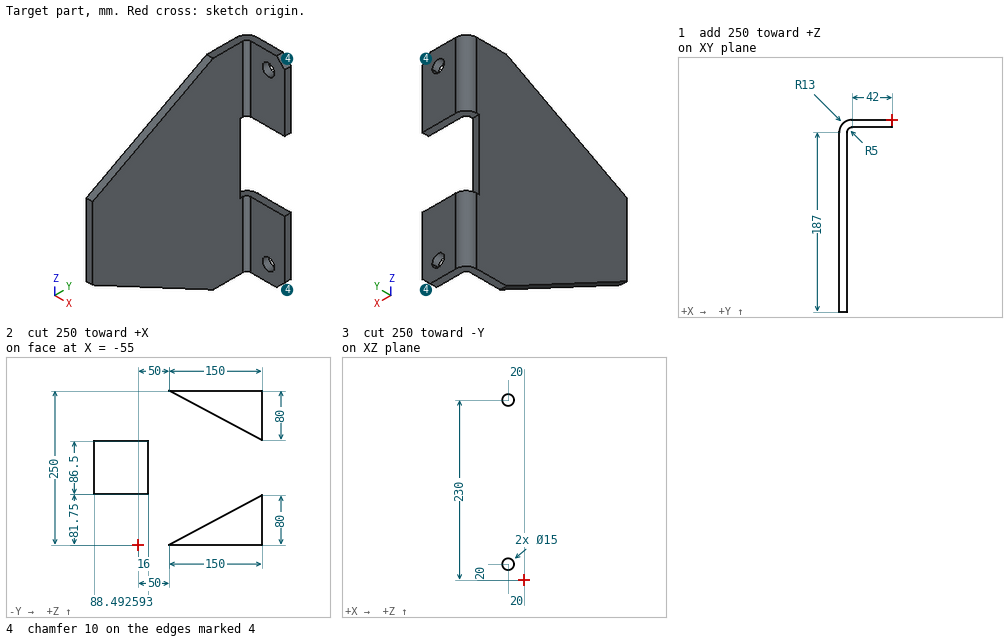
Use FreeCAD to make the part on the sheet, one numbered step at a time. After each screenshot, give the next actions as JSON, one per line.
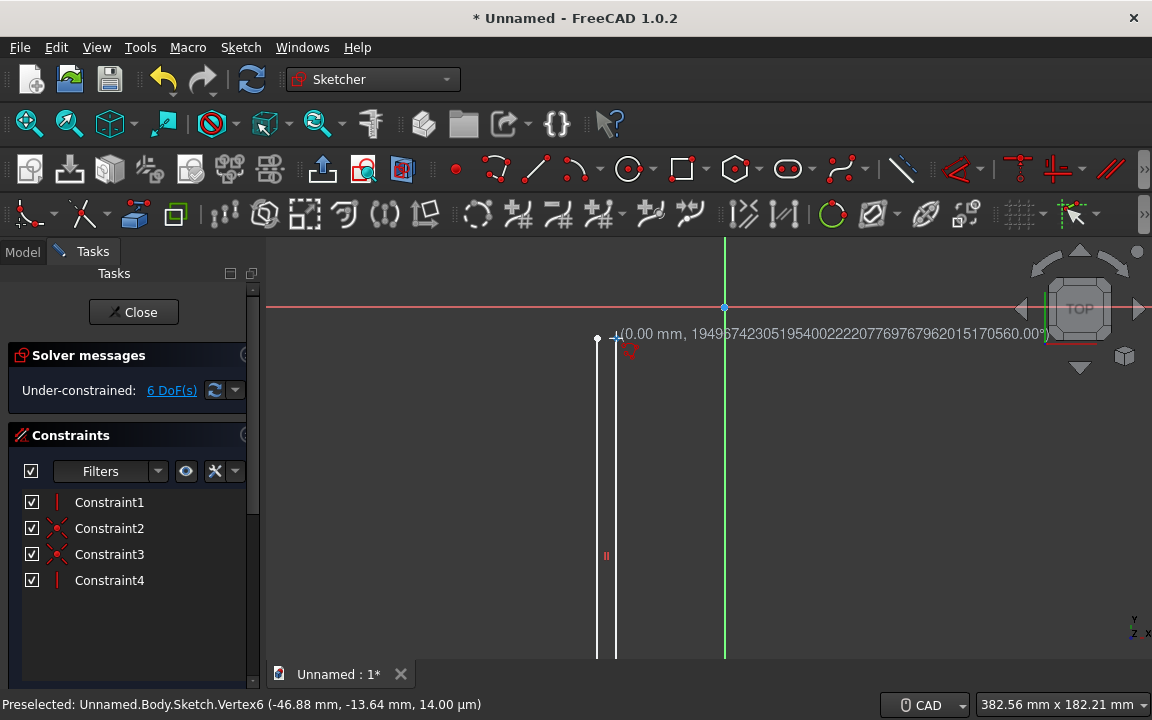
{"action": "left_click", "coordinate": [627, 326]}
{"action": "left_click", "coordinate": [725, 326]}
{"action": "left_click", "coordinate": [725, 307]}
{"action": "left_click", "coordinate": [627, 316]}
{"action": "right_click", "coordinate": [627, 316]}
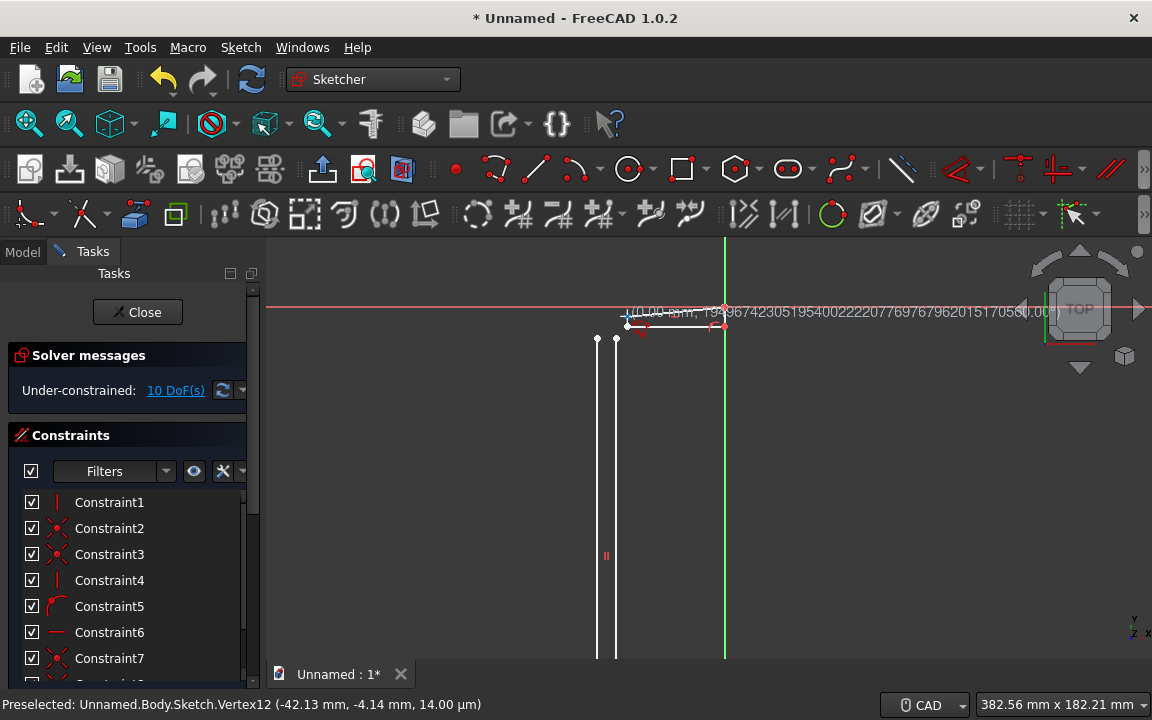
{"action": "left_click", "coordinate": [602, 170]}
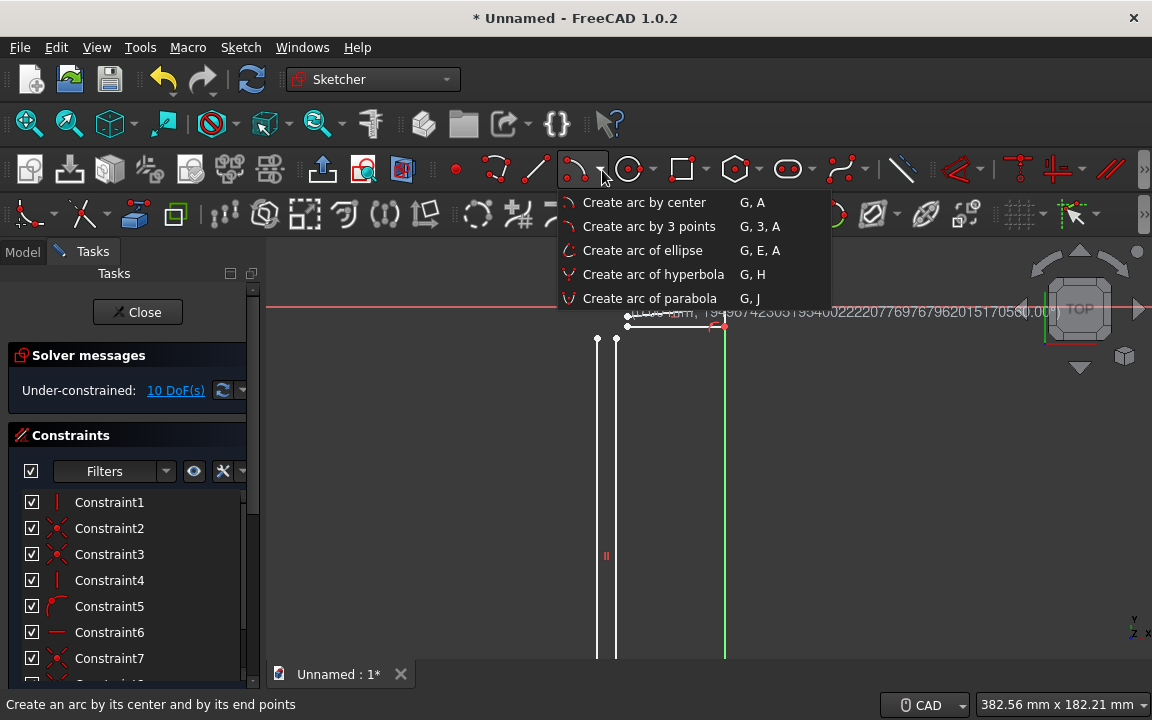
{"action": "left_click", "coordinate": [694, 226]}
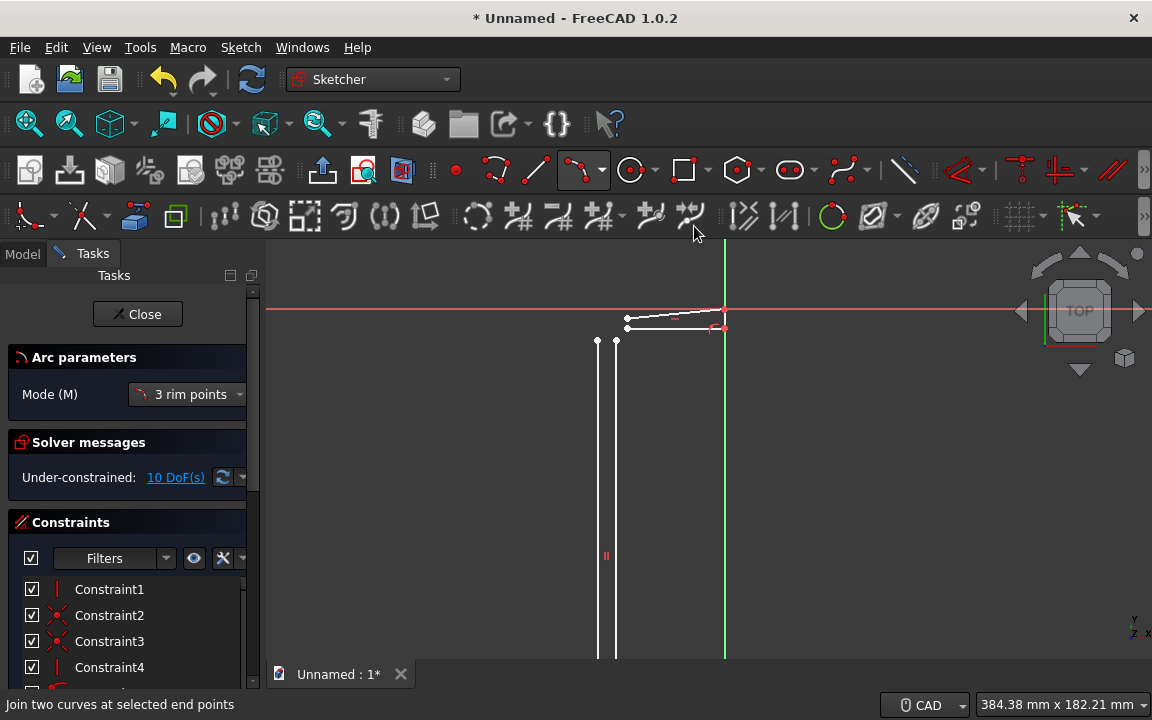
{"action": "left_click", "coordinate": [616, 341]}
{"action": "left_click", "coordinate": [627, 329]}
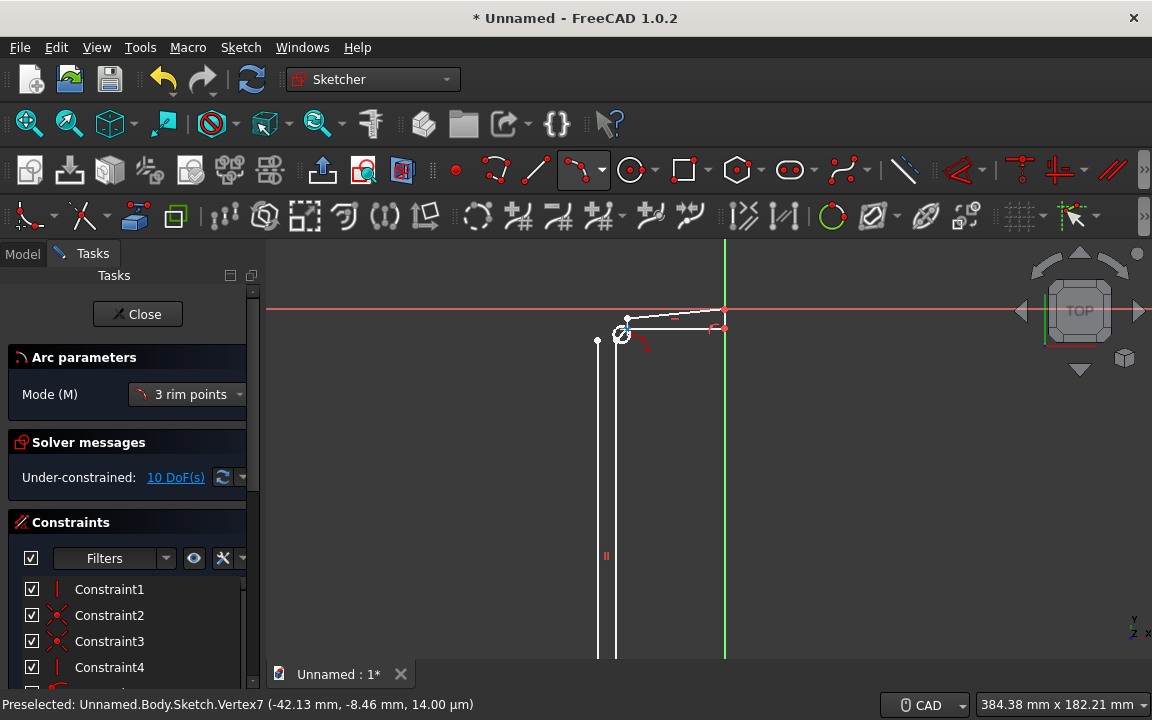
{"action": "scroll", "coordinate": [620, 331], "scroll_direction": "up", "scroll_amount": 8}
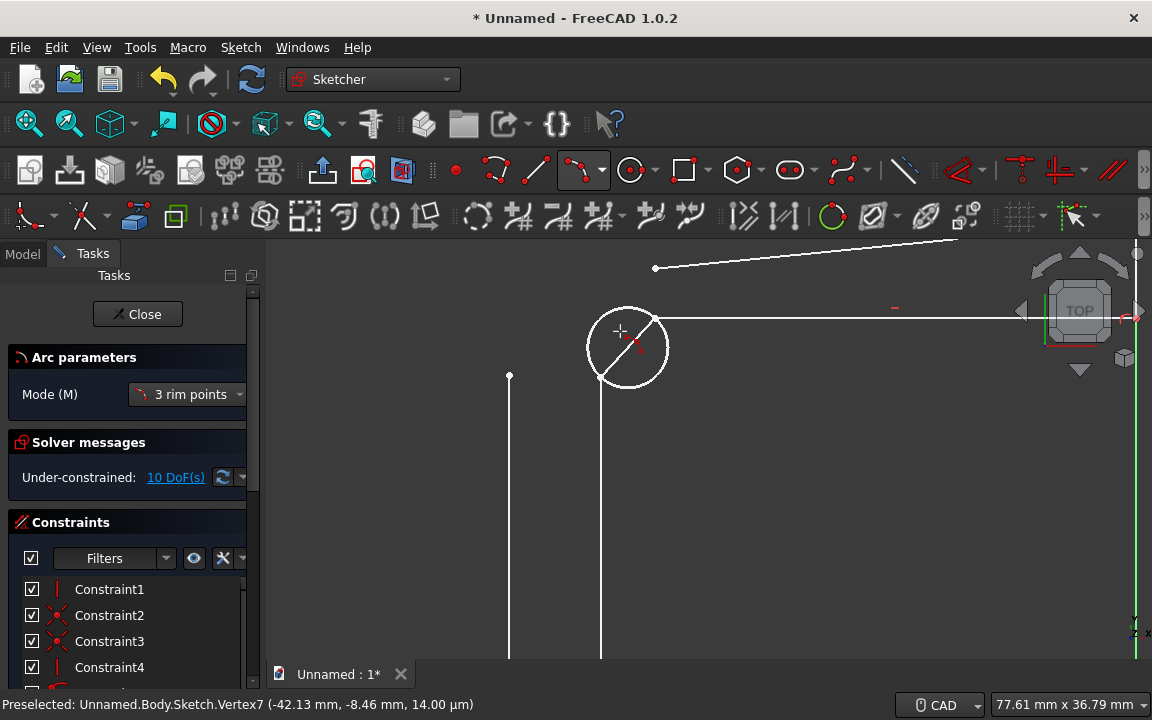
{"action": "left_click", "coordinate": [616, 330]}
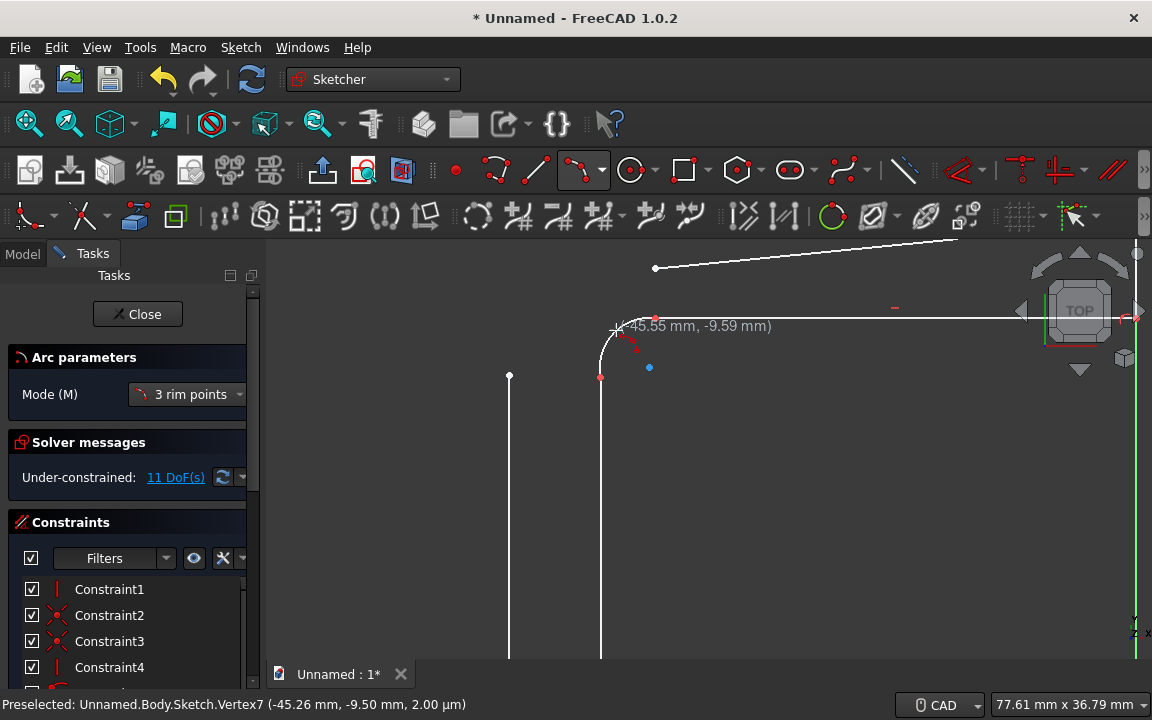
{"action": "scroll", "coordinate": [618, 335], "scroll_direction": "down", "scroll_amount": 11}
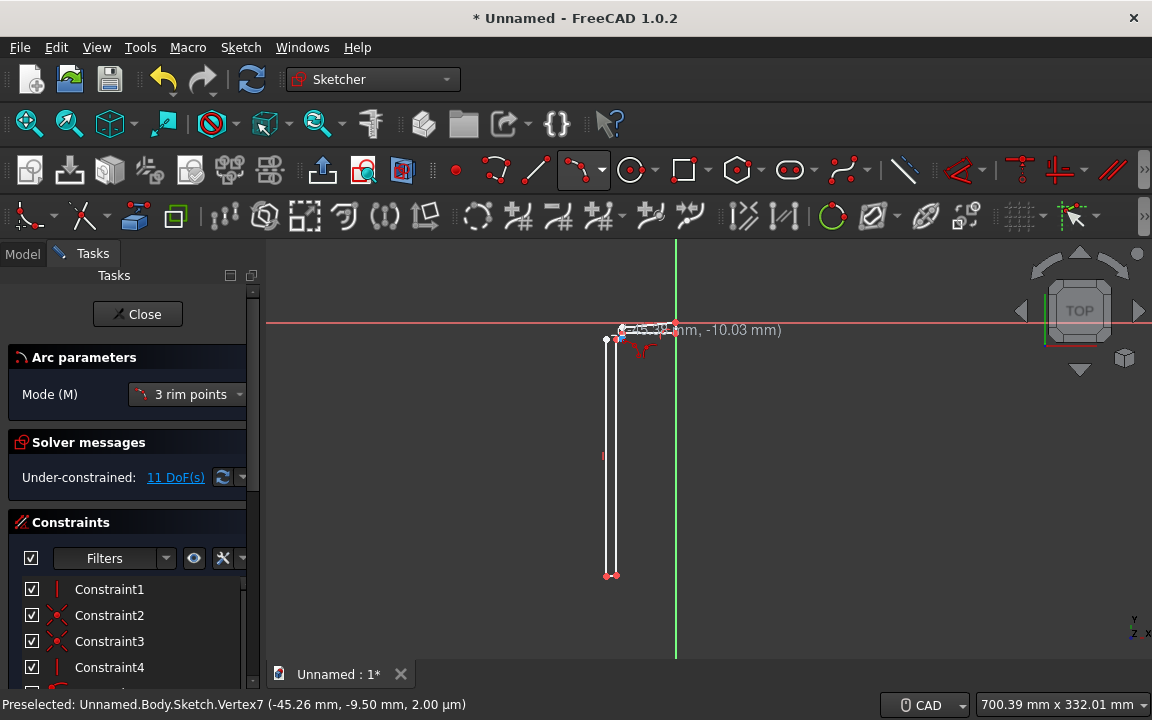
{"action": "scroll", "coordinate": [623, 323], "scroll_direction": "up", "scroll_amount": 3}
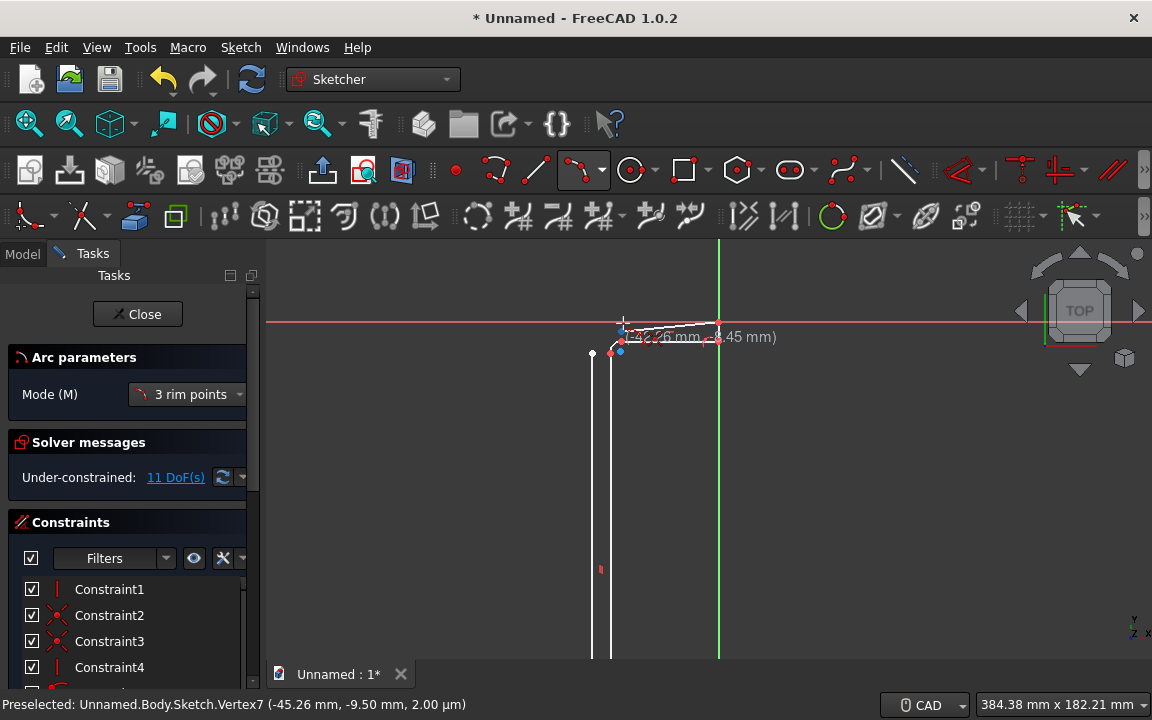
{"action": "left_click", "coordinate": [622, 332]}
{"action": "left_click", "coordinate": [592, 353]}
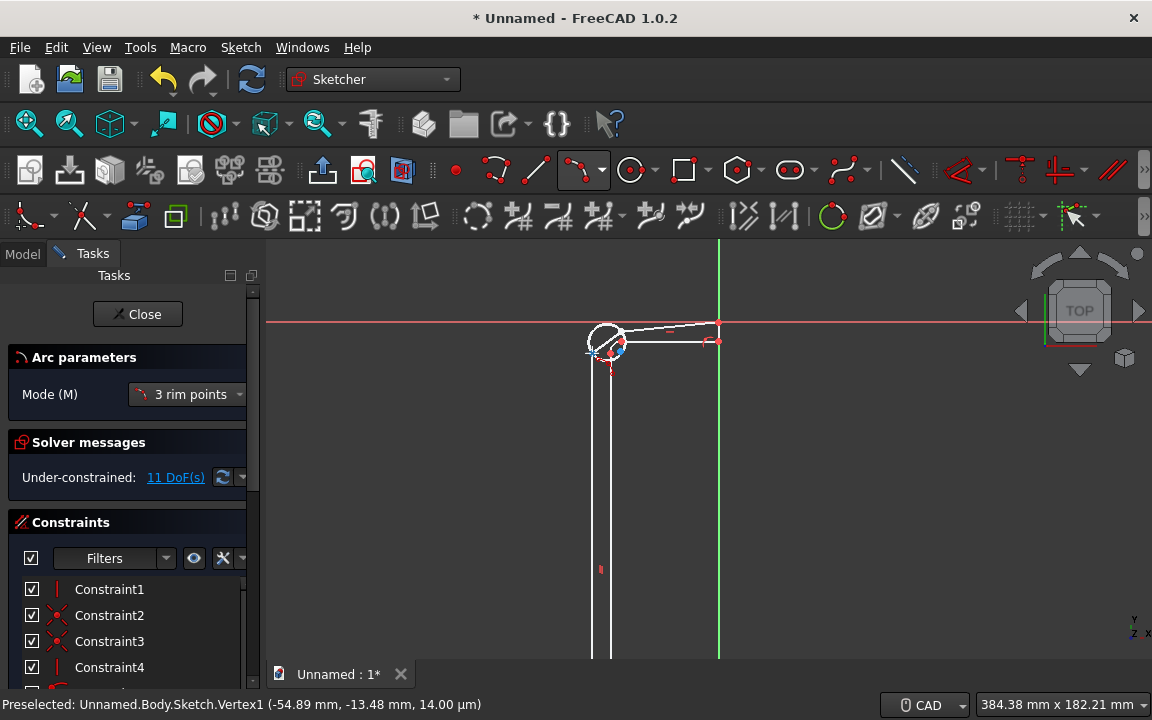
{"action": "scroll", "coordinate": [601, 331], "scroll_direction": "up", "scroll_amount": 3}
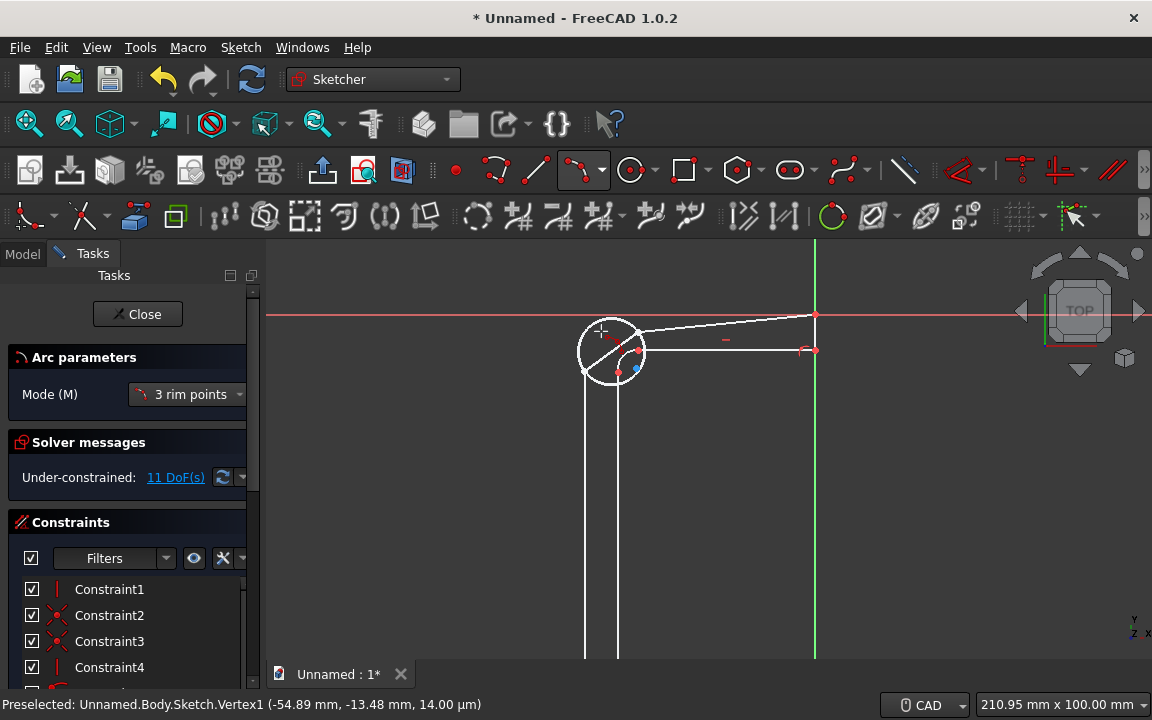
{"action": "left_click", "coordinate": [600, 331]}
{"action": "key", "text": "Escape"}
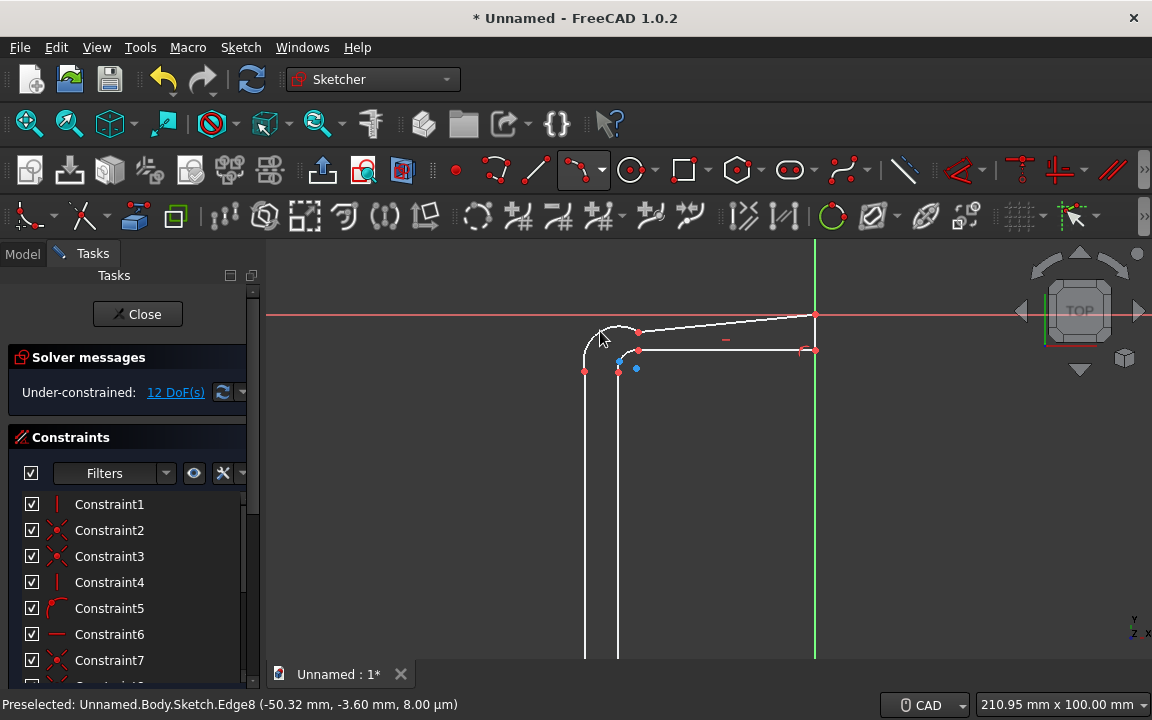
{"action": "left_click", "coordinate": [585, 607]}